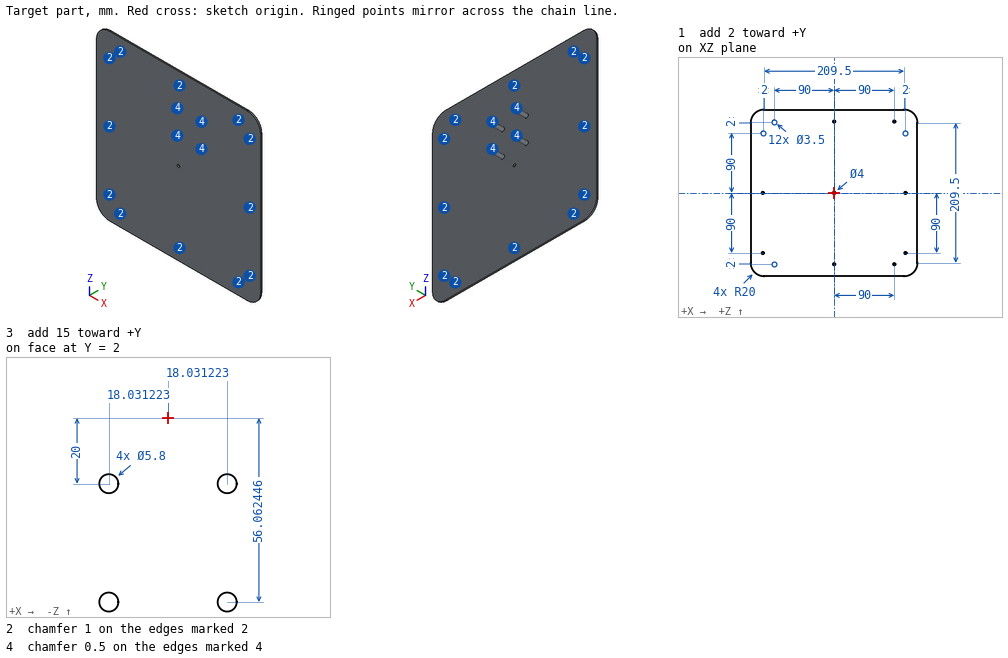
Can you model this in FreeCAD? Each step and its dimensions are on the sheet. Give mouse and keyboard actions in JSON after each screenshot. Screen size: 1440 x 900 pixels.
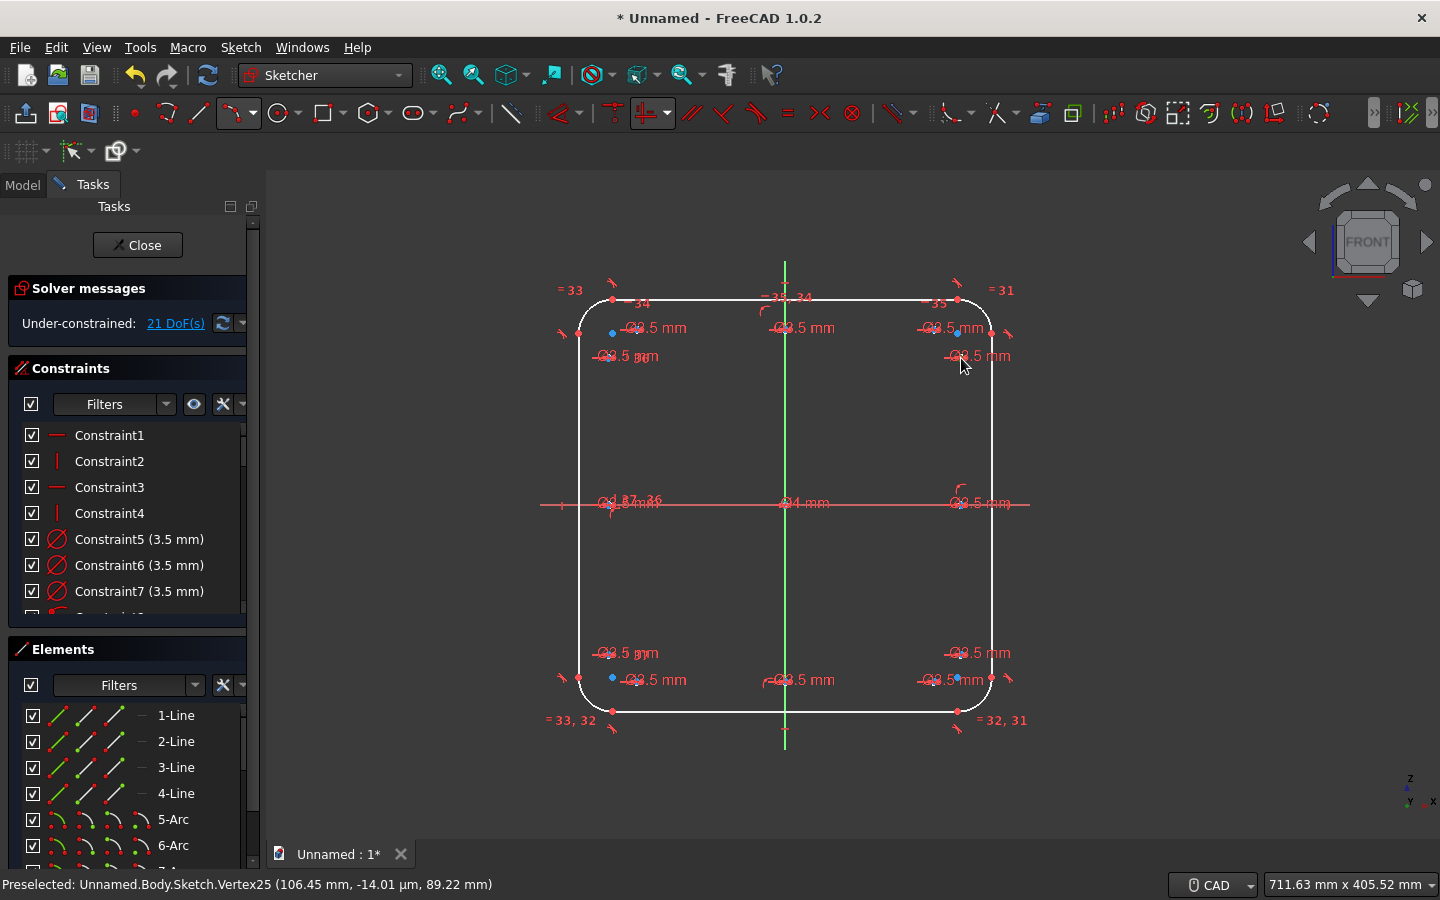
{"action": "left_click", "coordinate": [961, 505]}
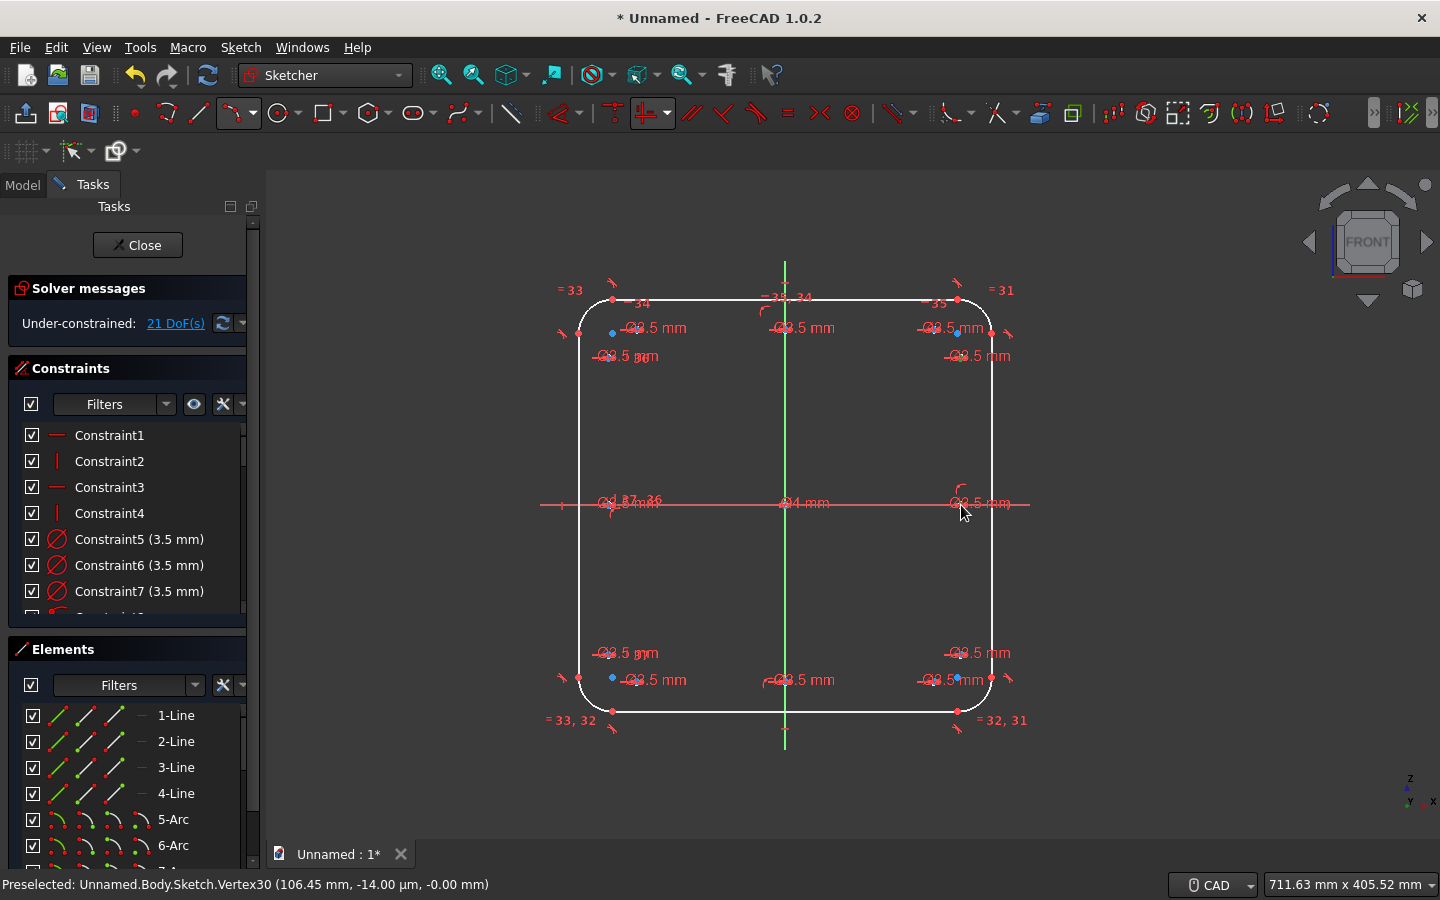
{"action": "key", "text": "v"}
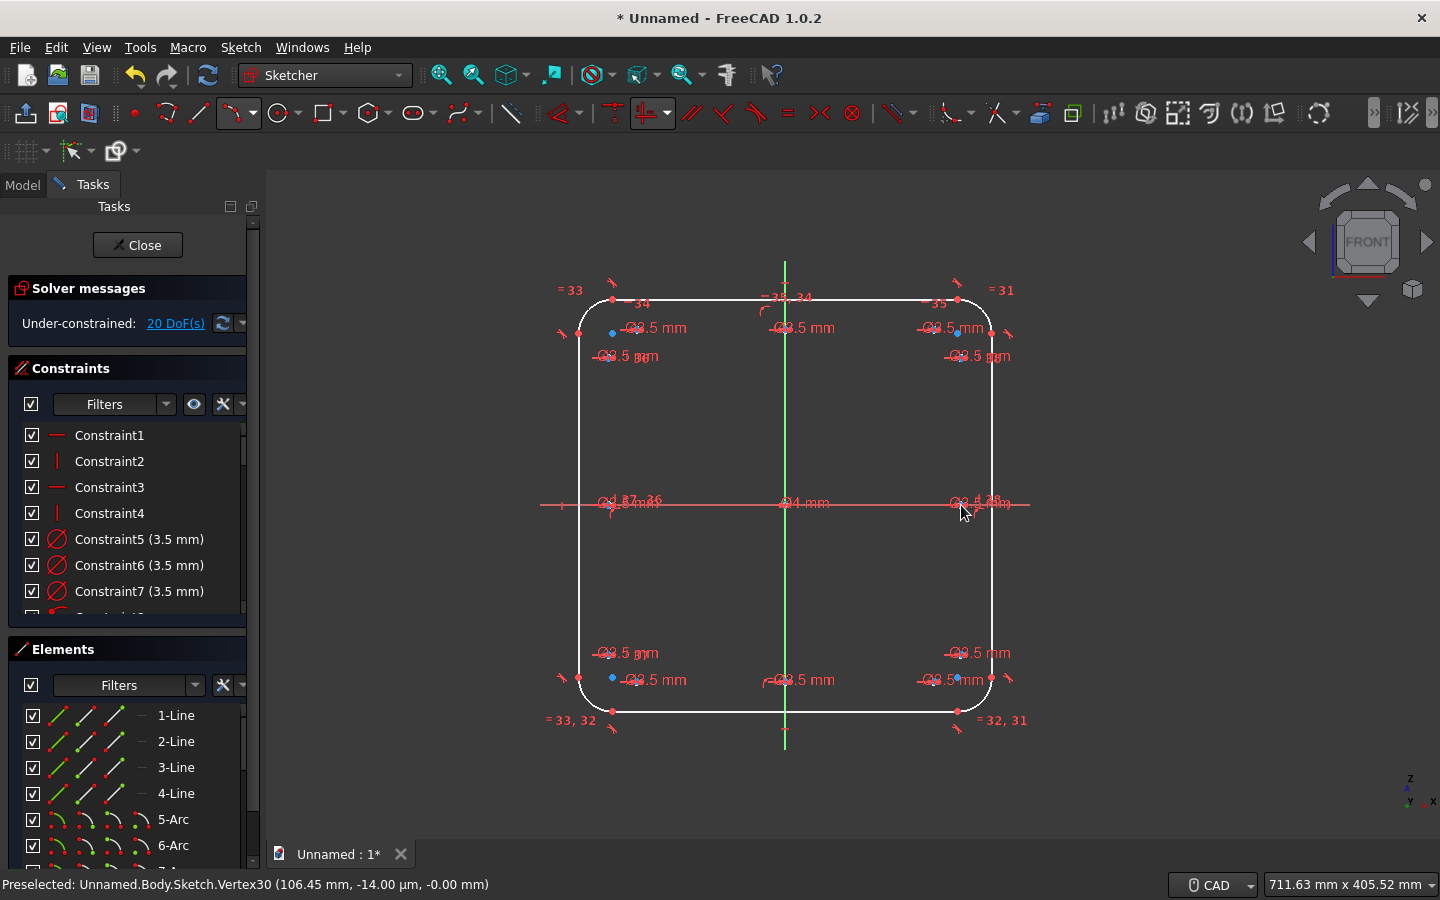
{"action": "left_click", "coordinate": [637, 682]}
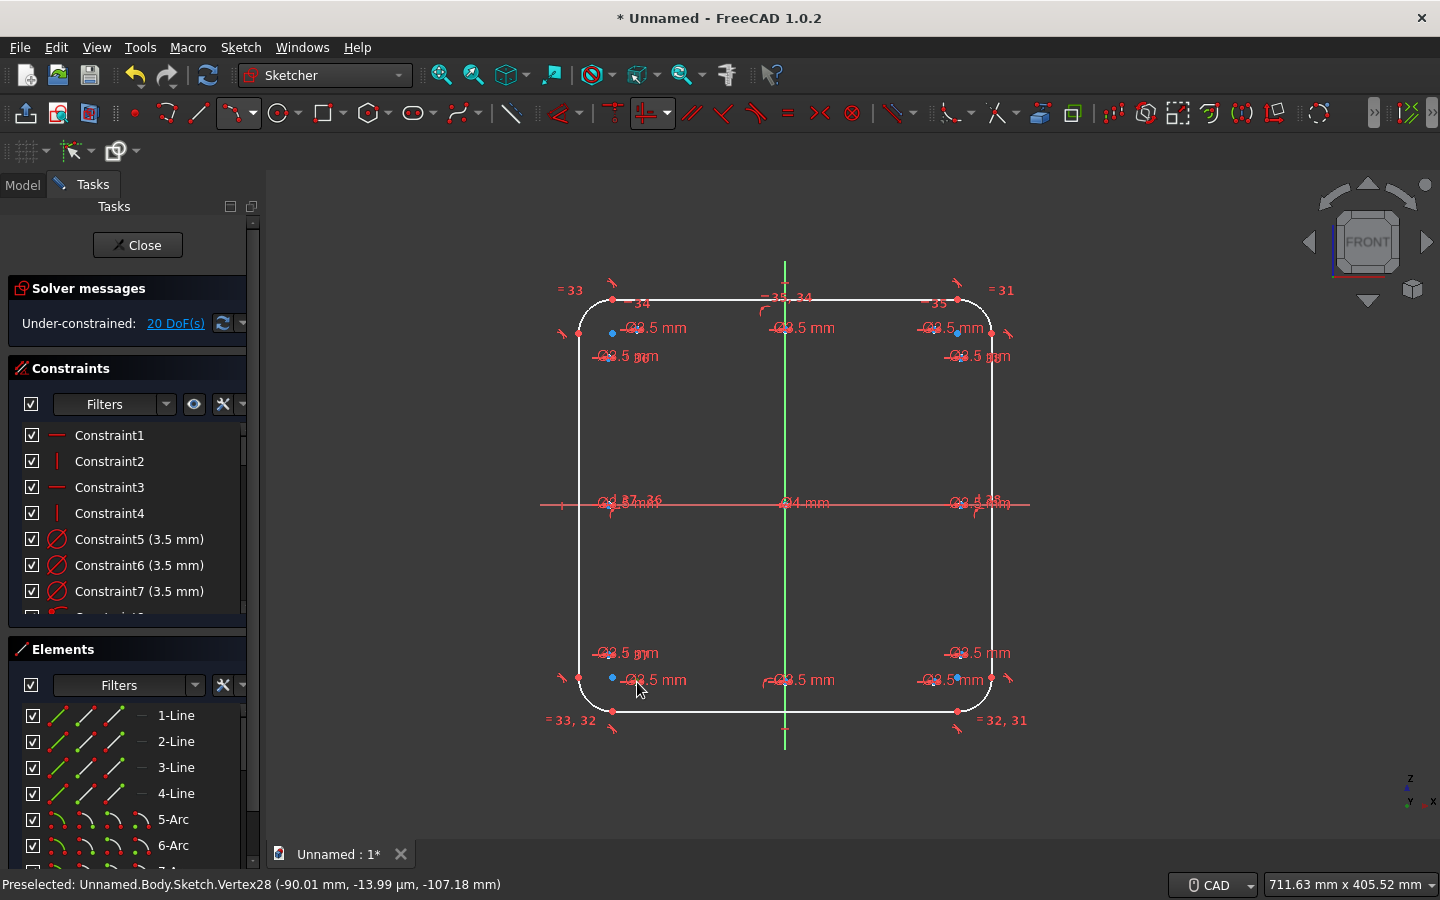
{"action": "left_click", "coordinate": [785, 682]}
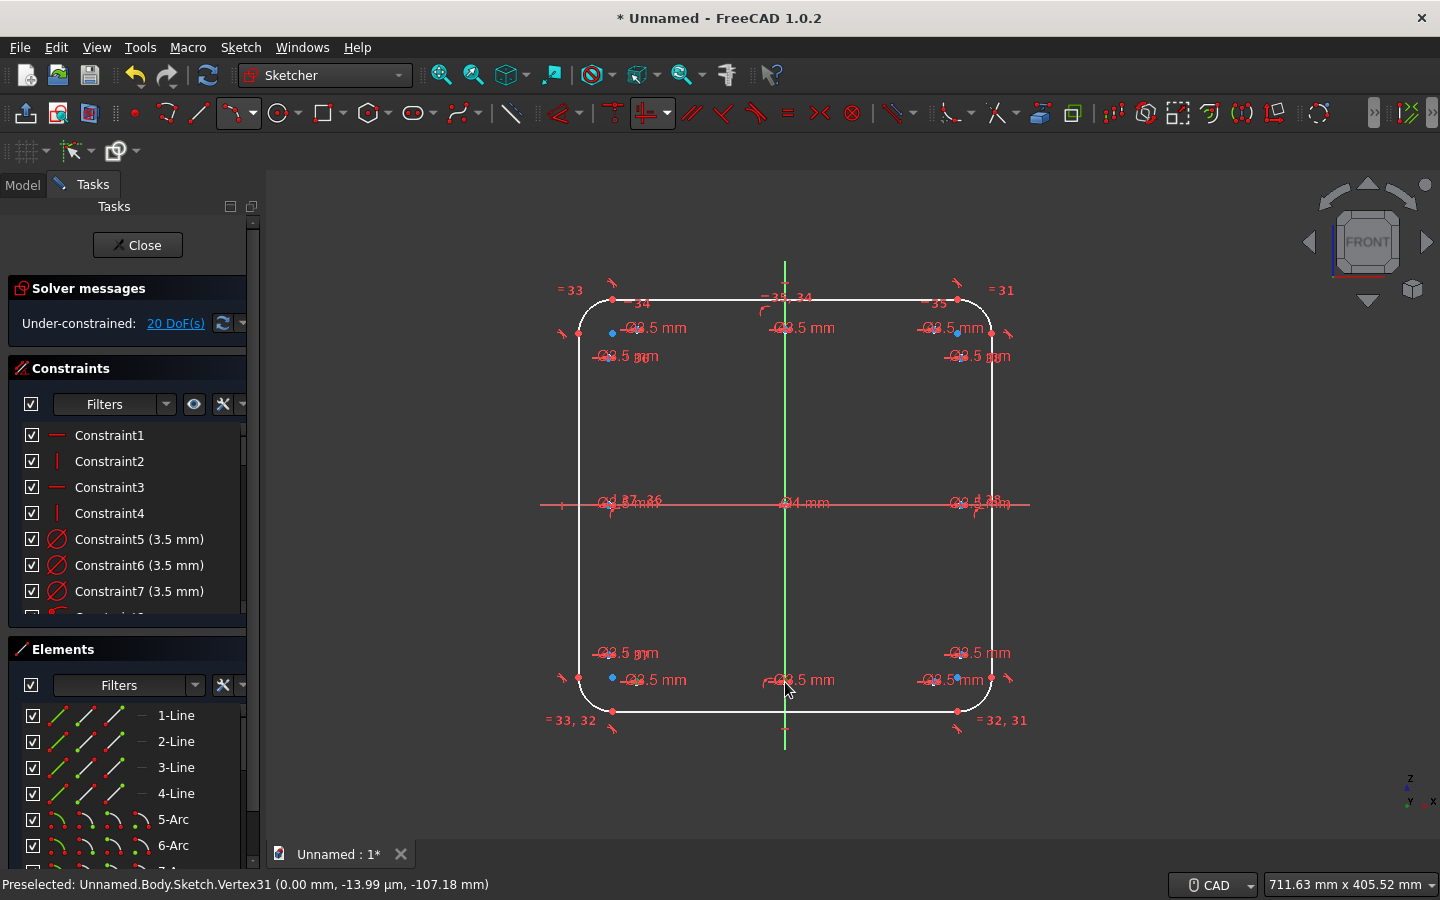
{"action": "key", "text": "h"}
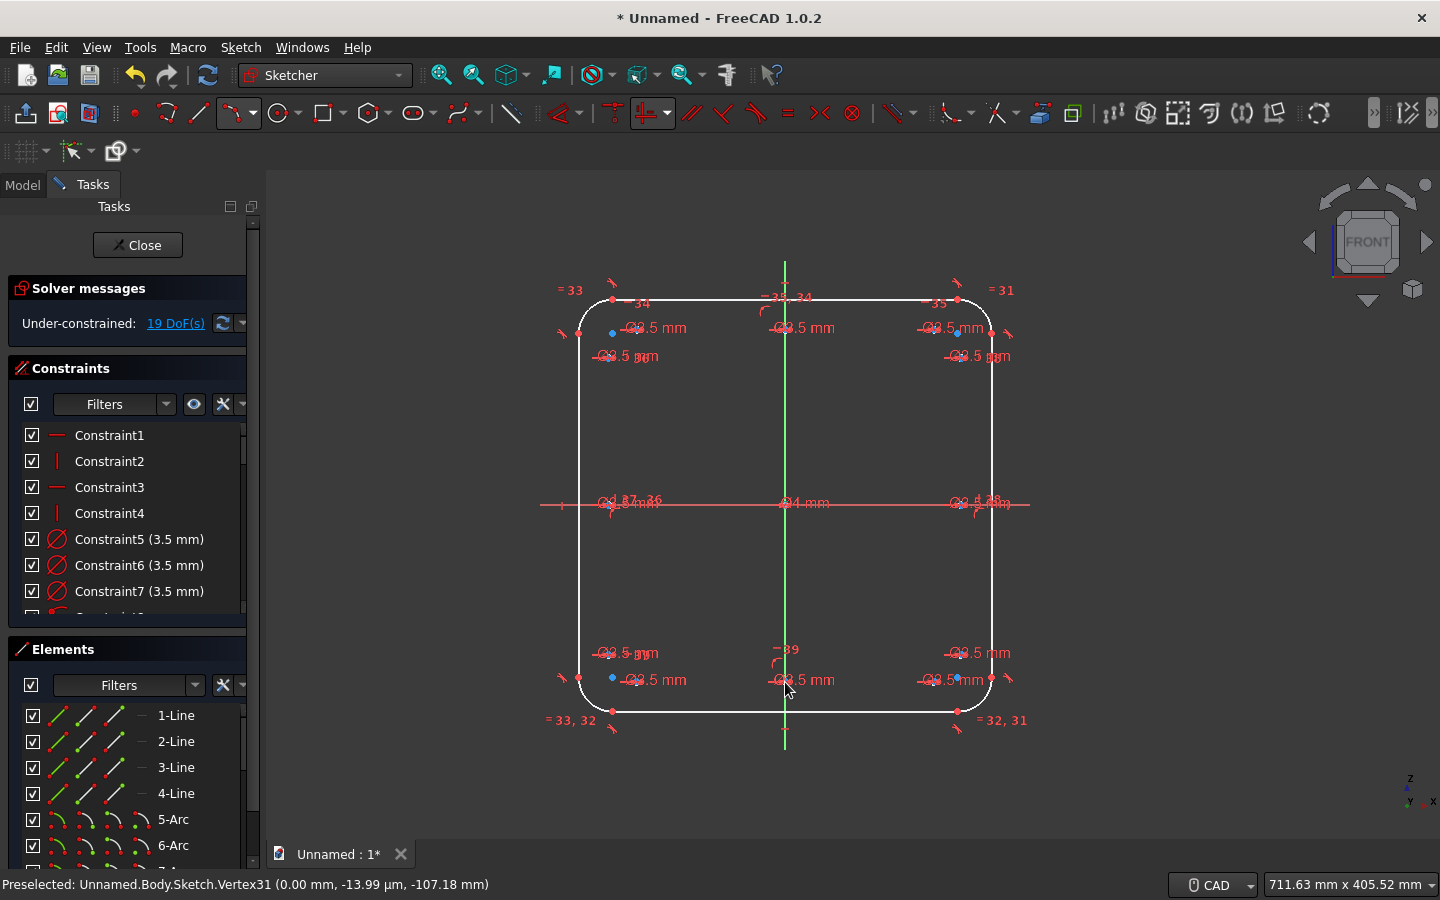
{"action": "left_click", "coordinate": [961, 505]}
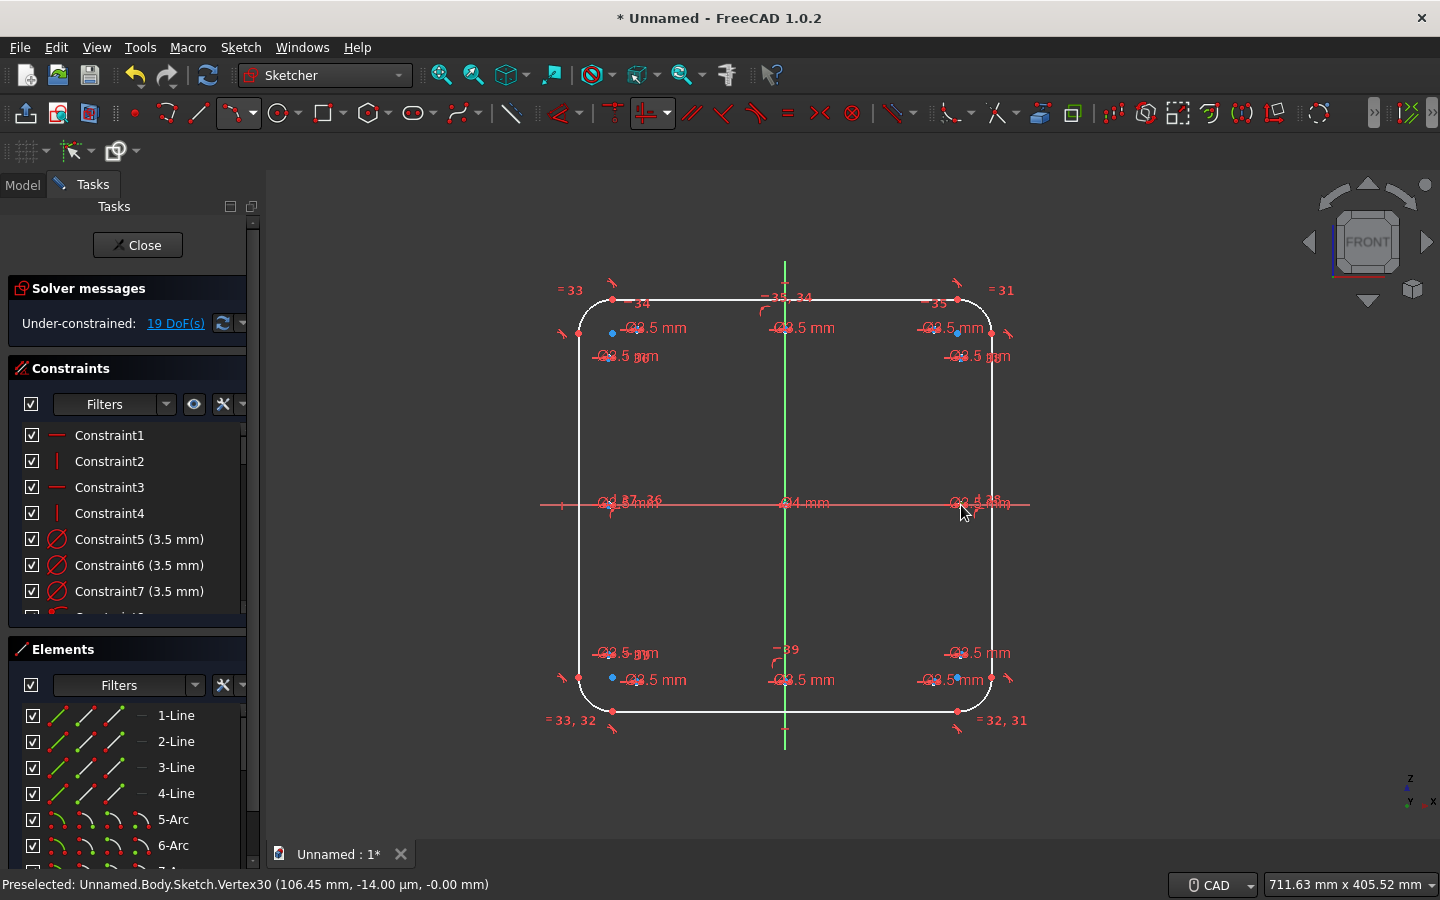
{"action": "left_click", "coordinate": [961, 655]}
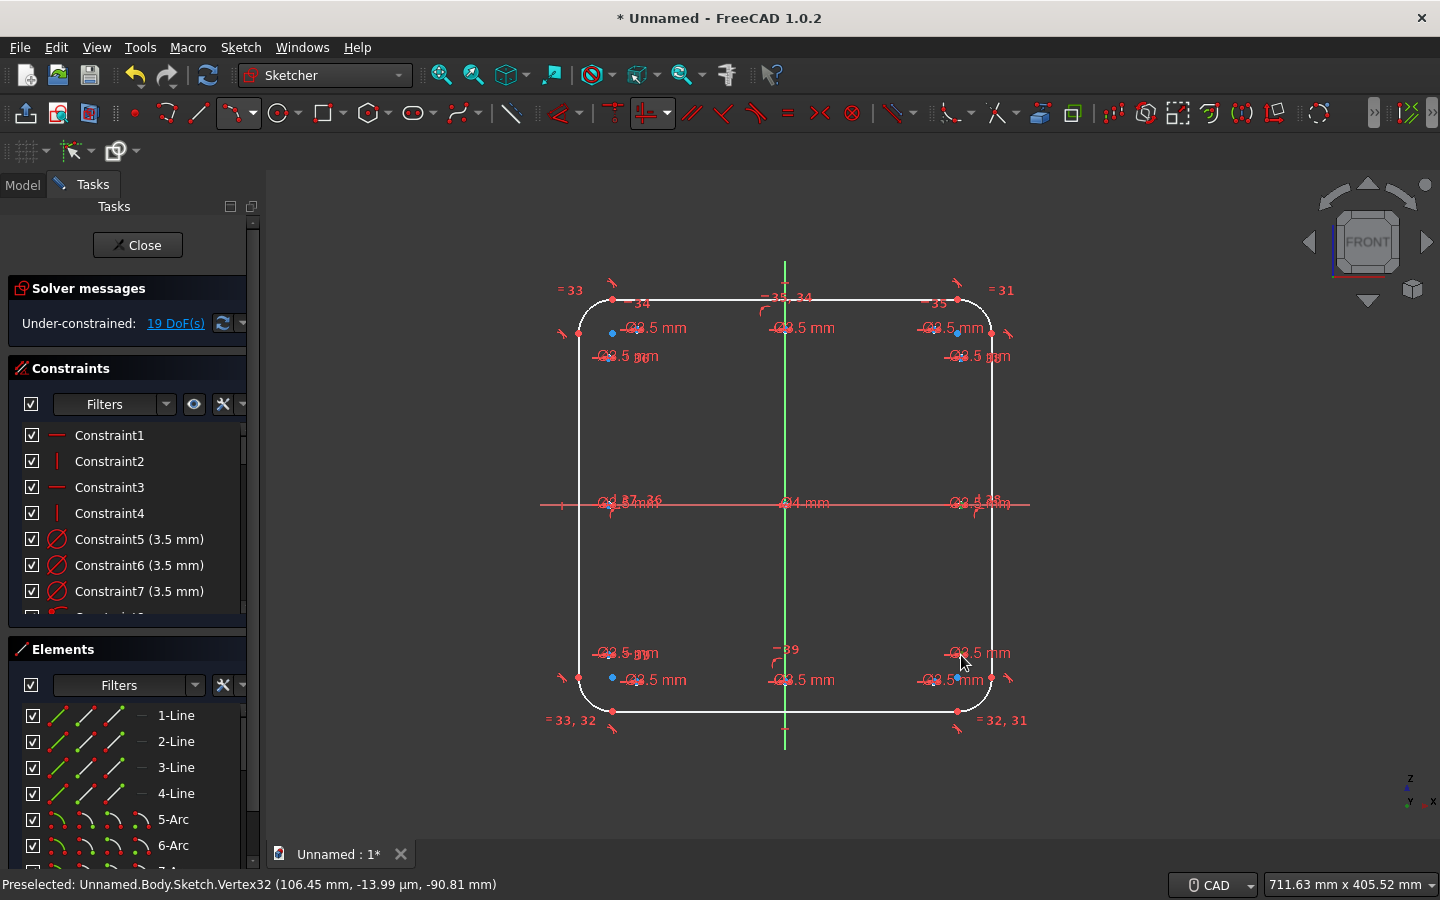
{"action": "key", "text": "v"}